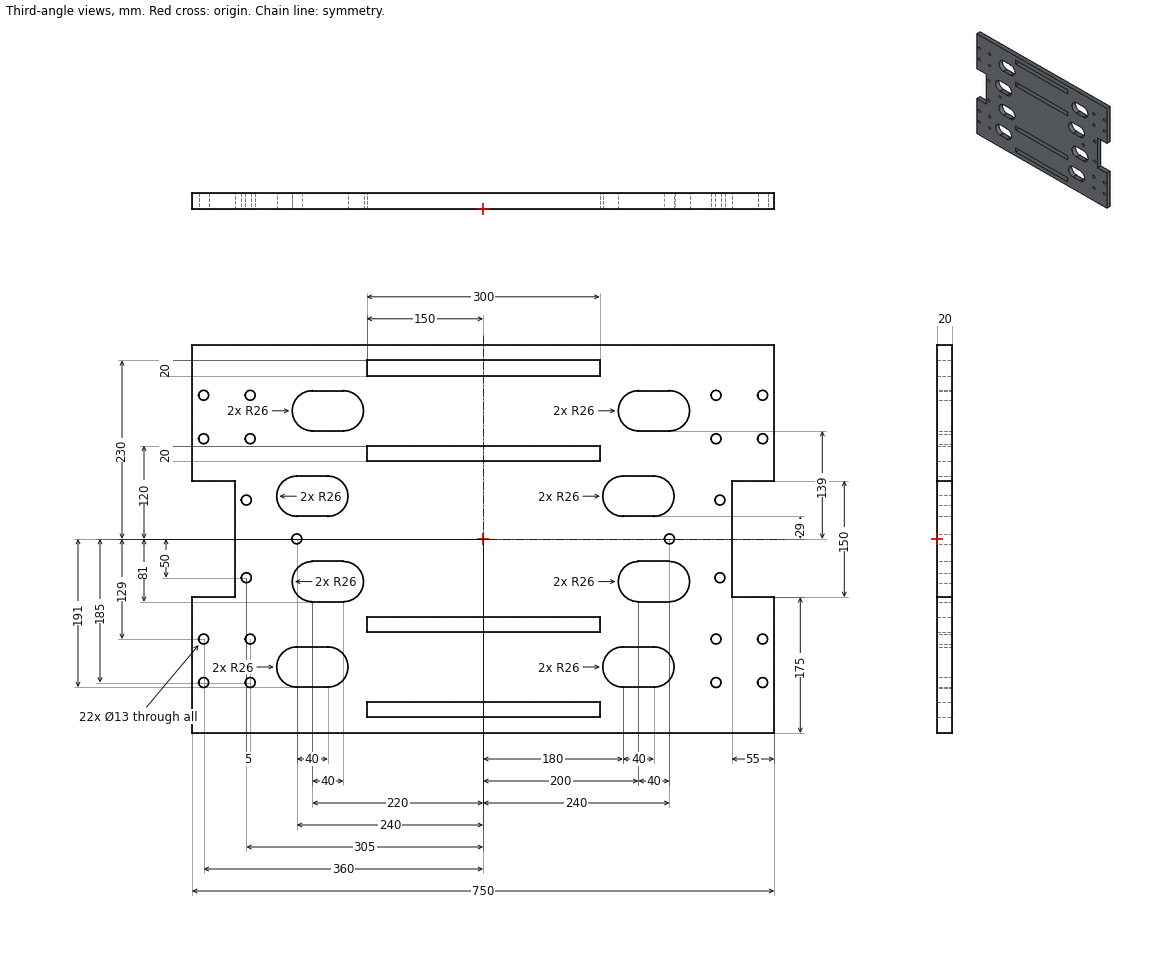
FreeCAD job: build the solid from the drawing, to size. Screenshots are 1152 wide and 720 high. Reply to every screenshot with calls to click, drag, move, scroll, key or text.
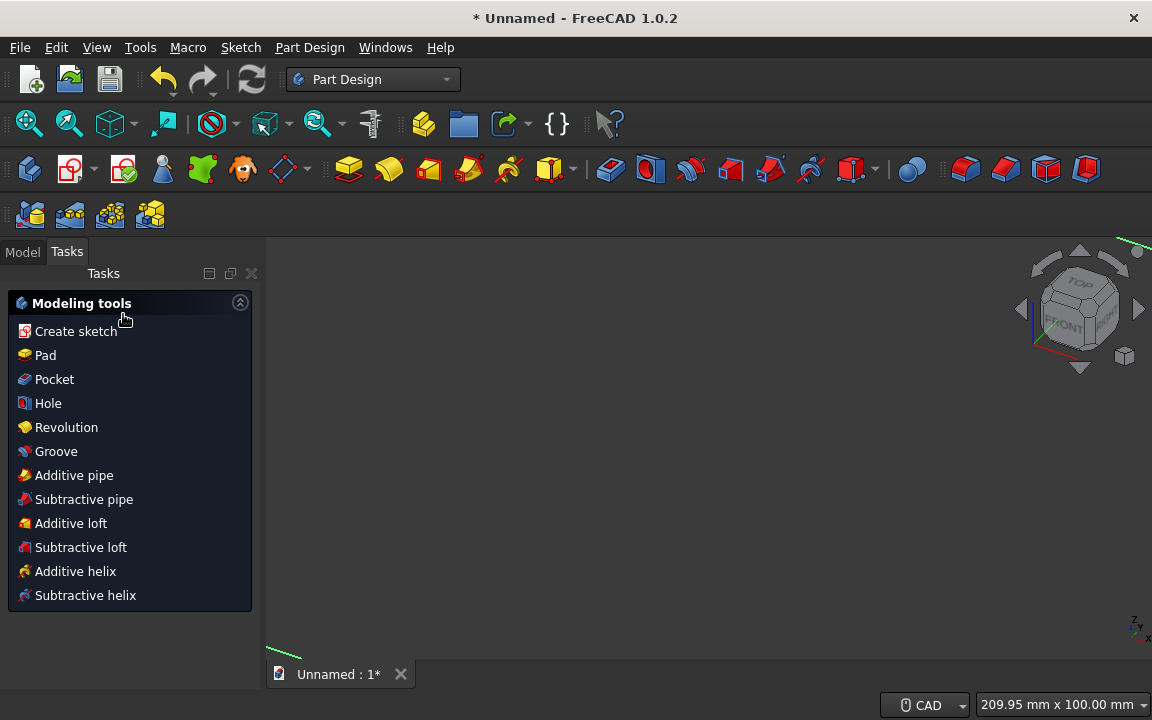
click(350, 170)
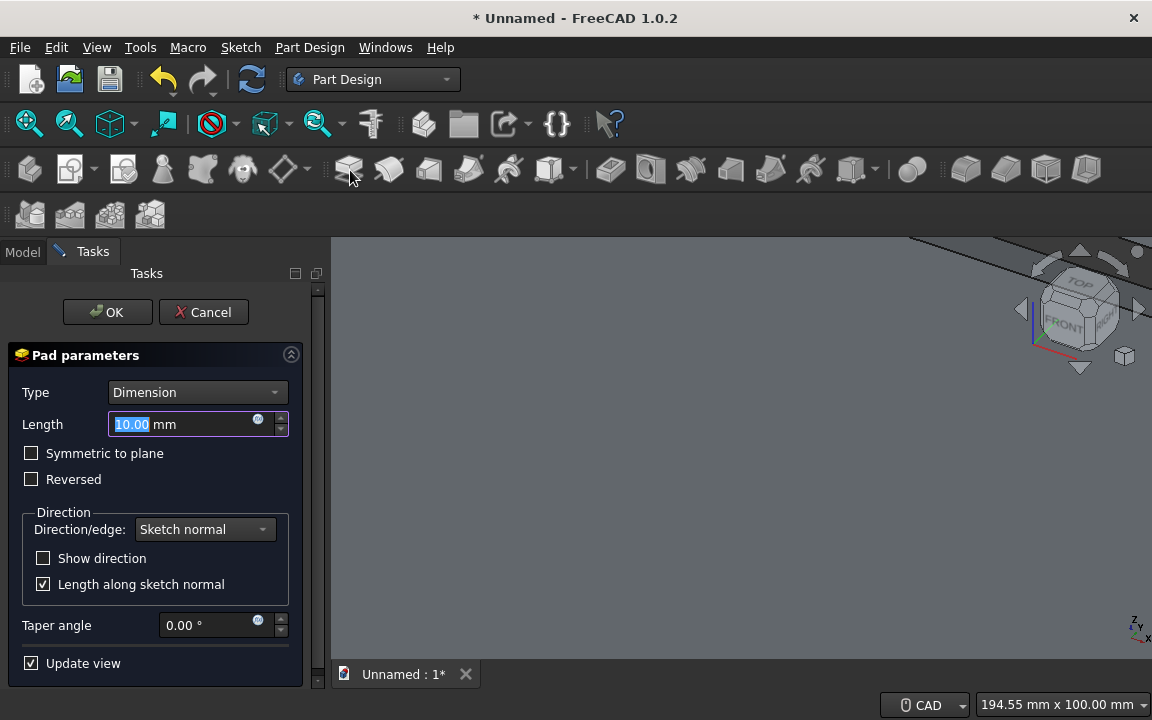
text(20)
key(Tab)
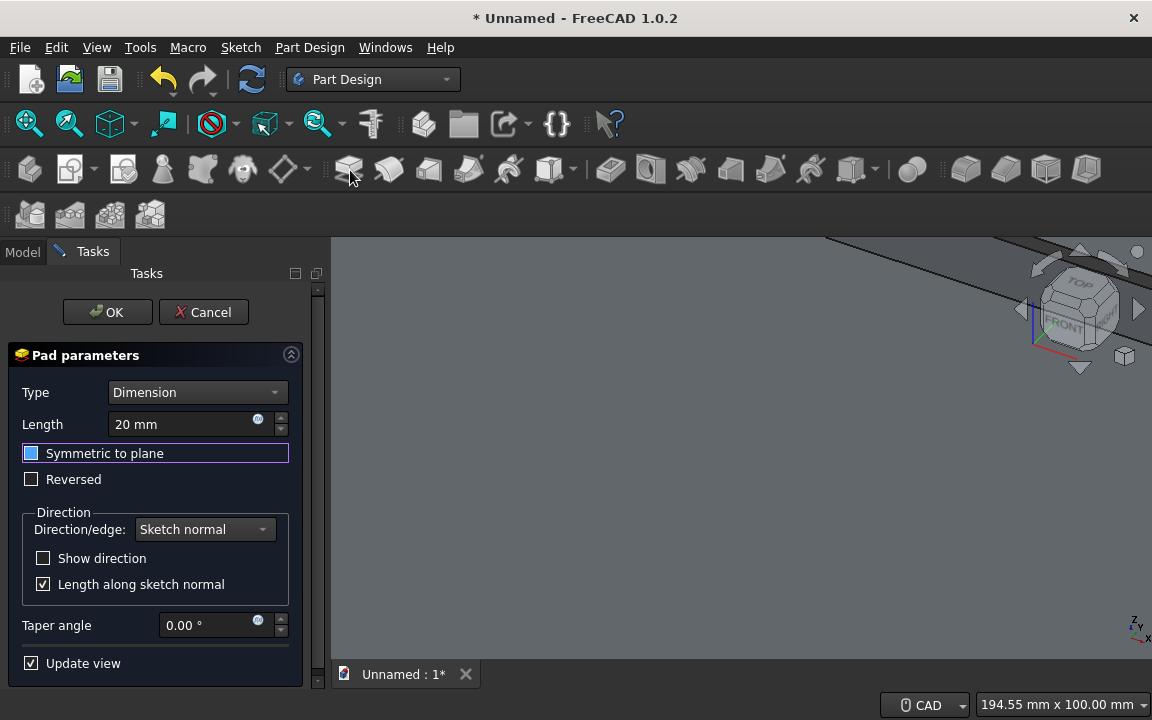
click(30, 479)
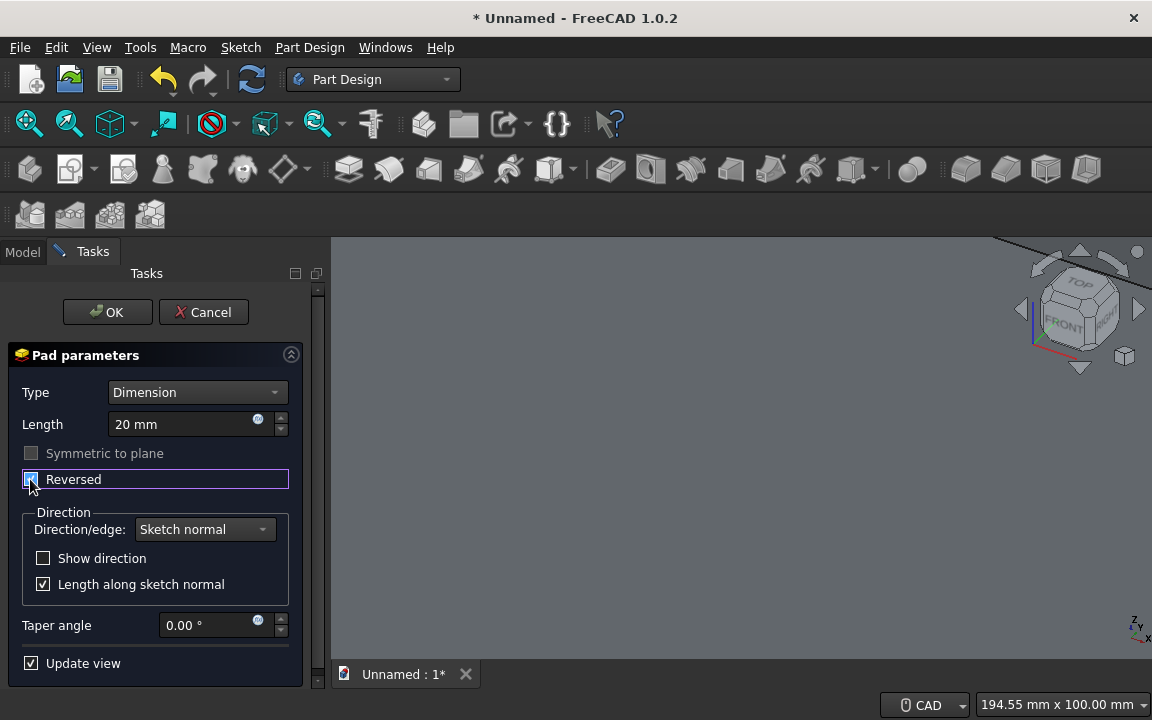
click(108, 312)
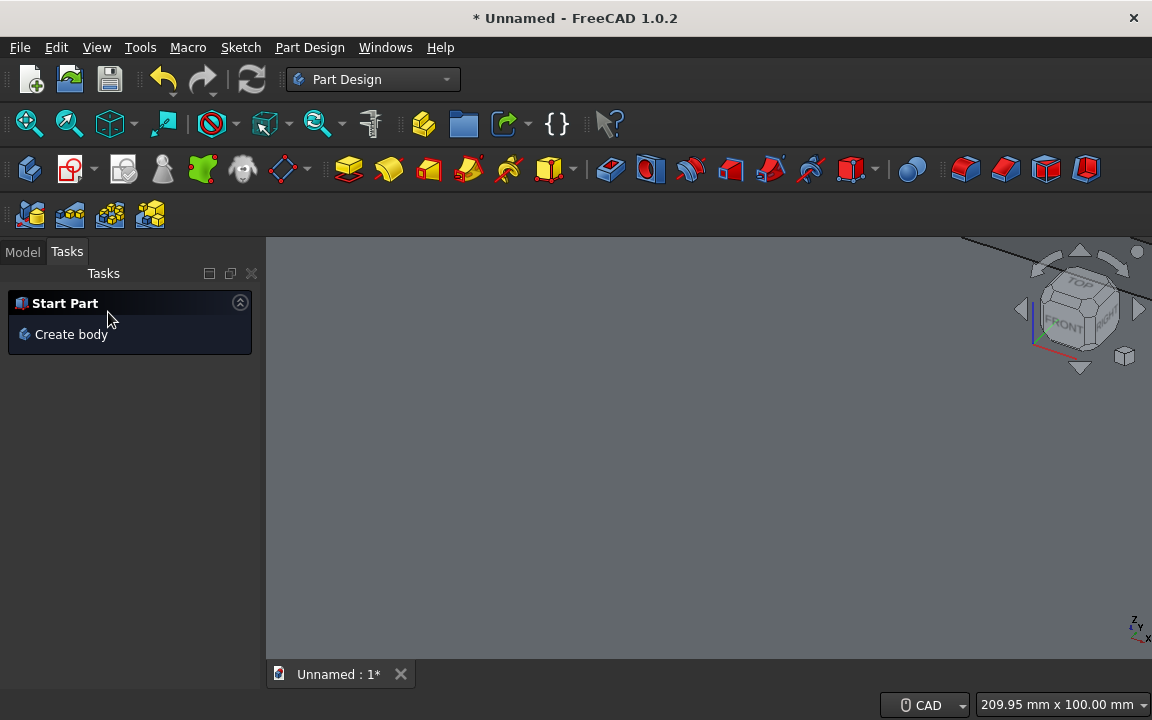
click(30, 124)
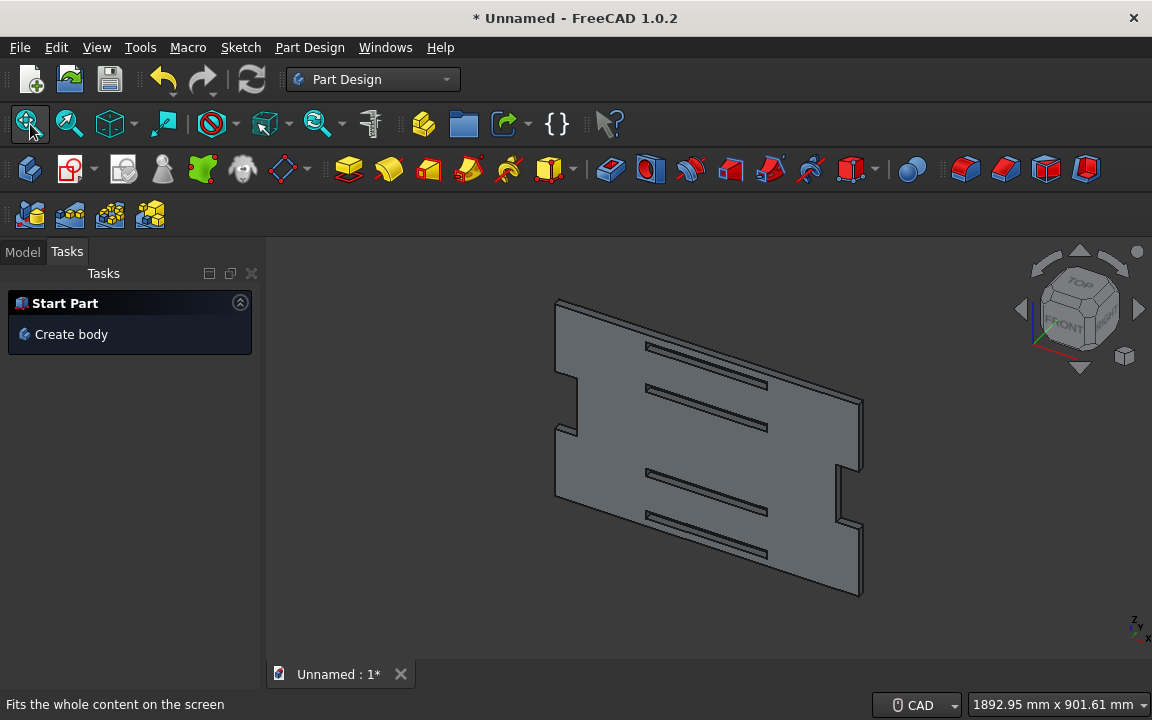
key(4)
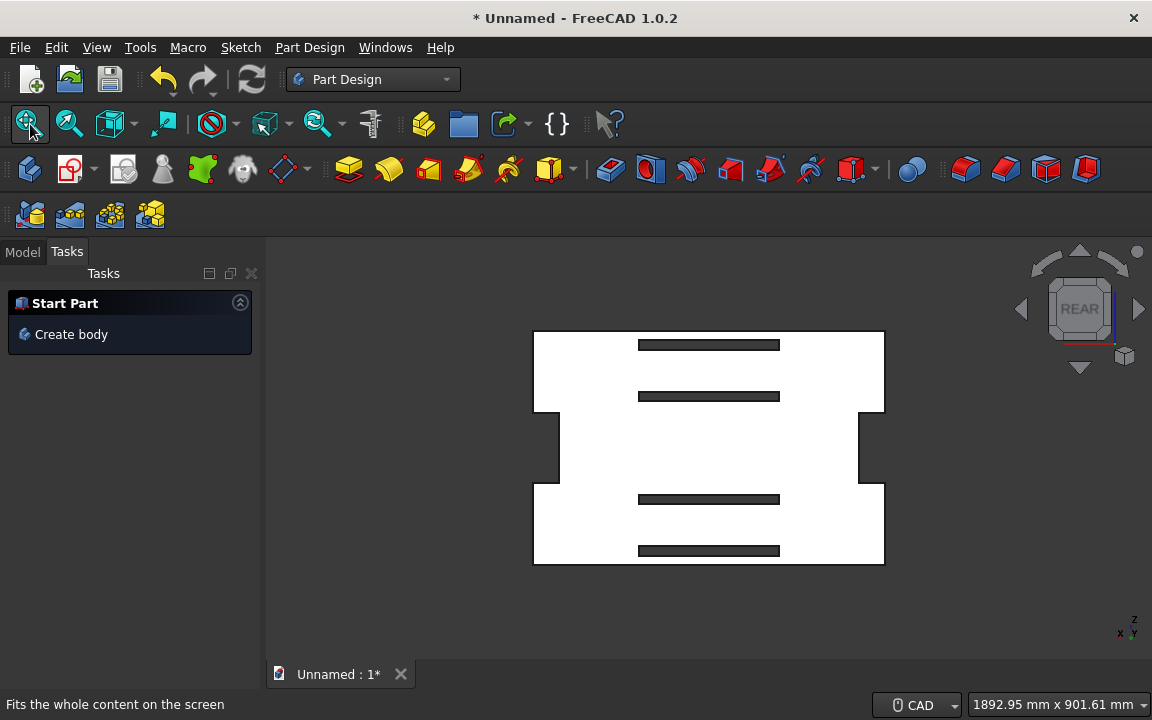
click(809, 447)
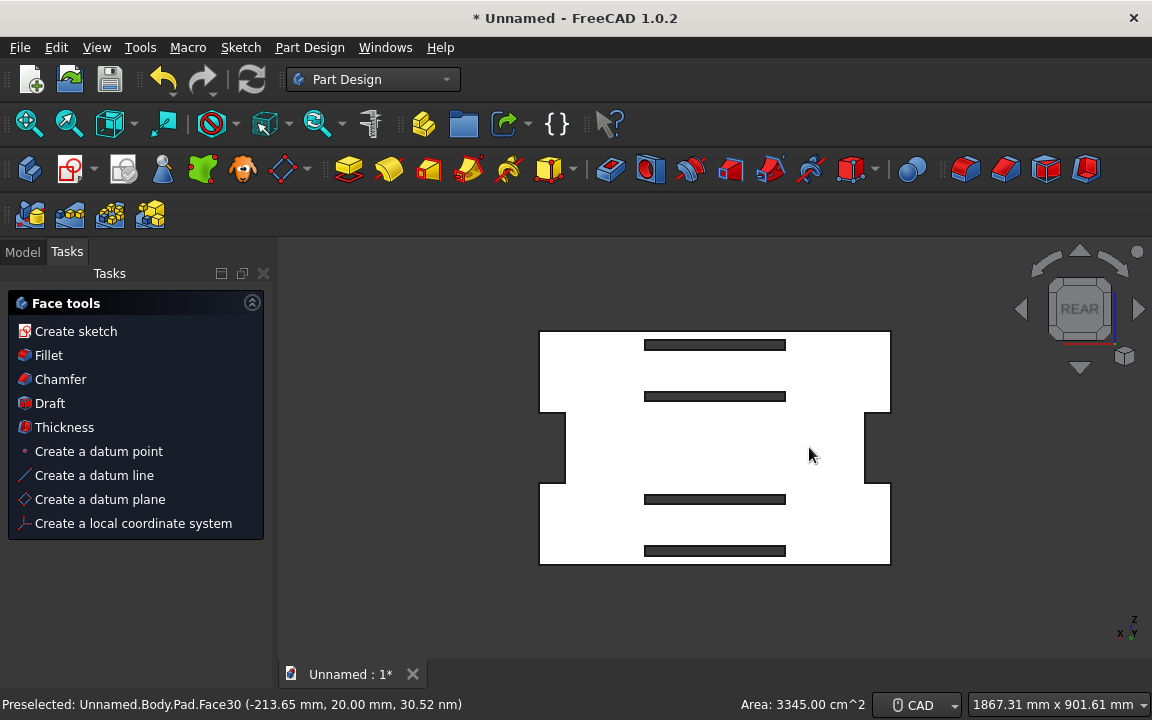
click(70, 170)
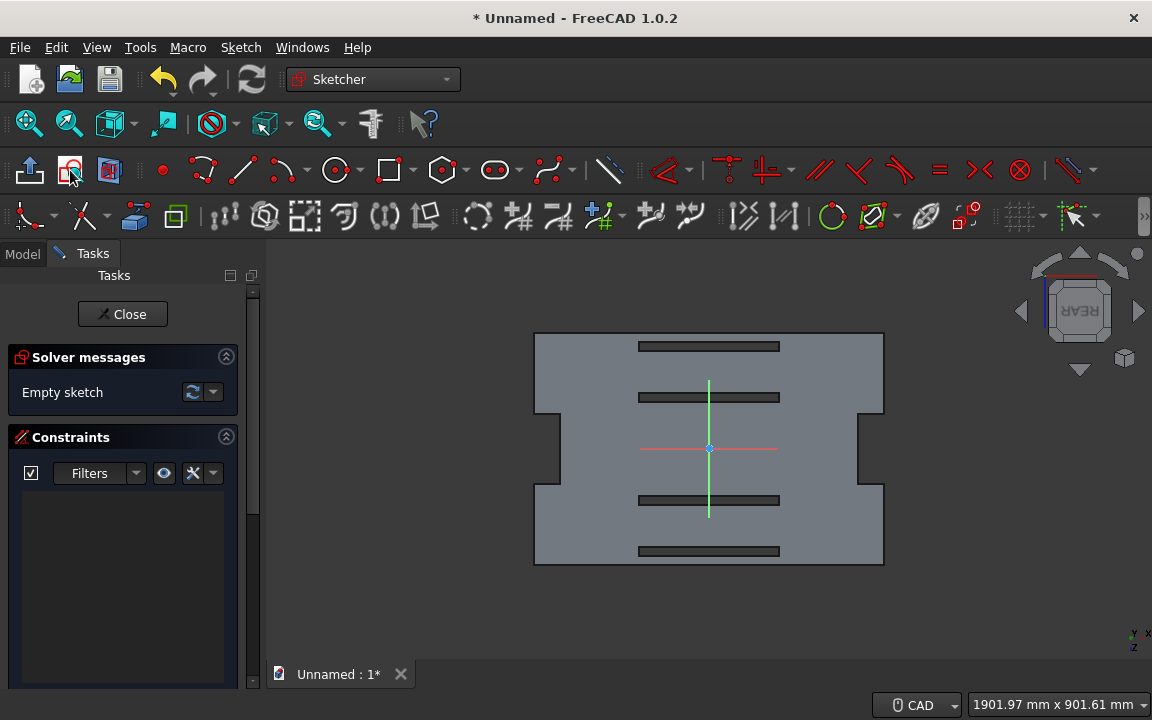
scroll(848, 449, up, 2)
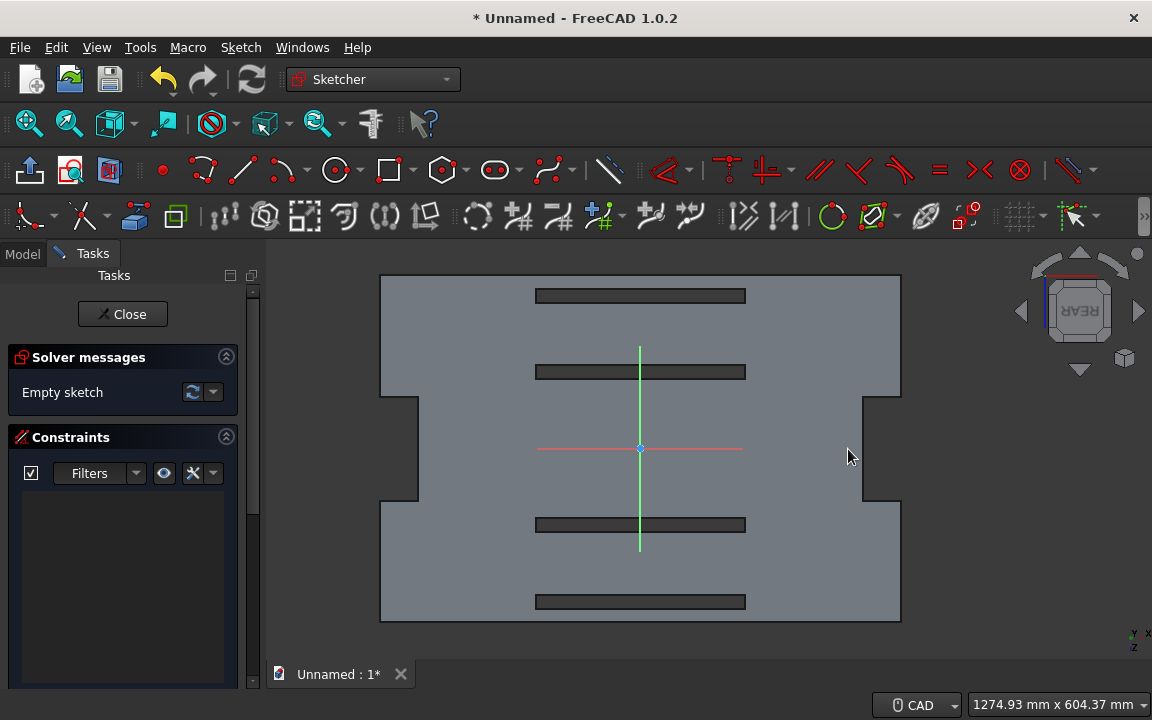
click(336, 170)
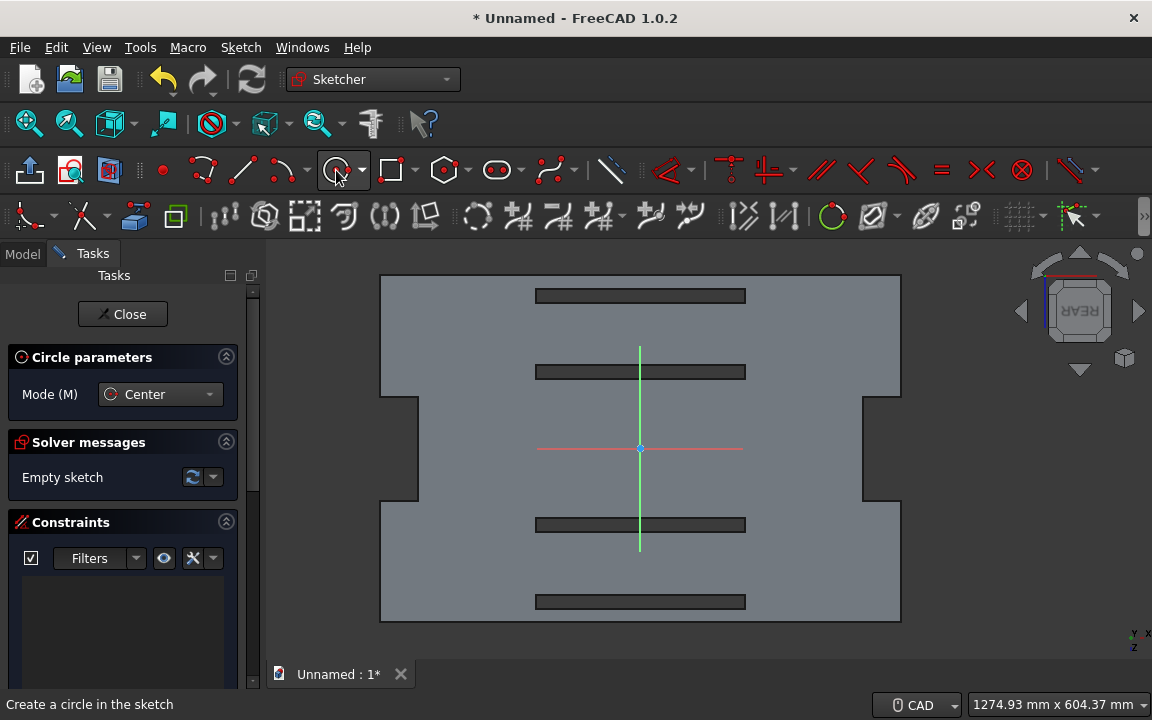
scroll(390, 359, up, 9)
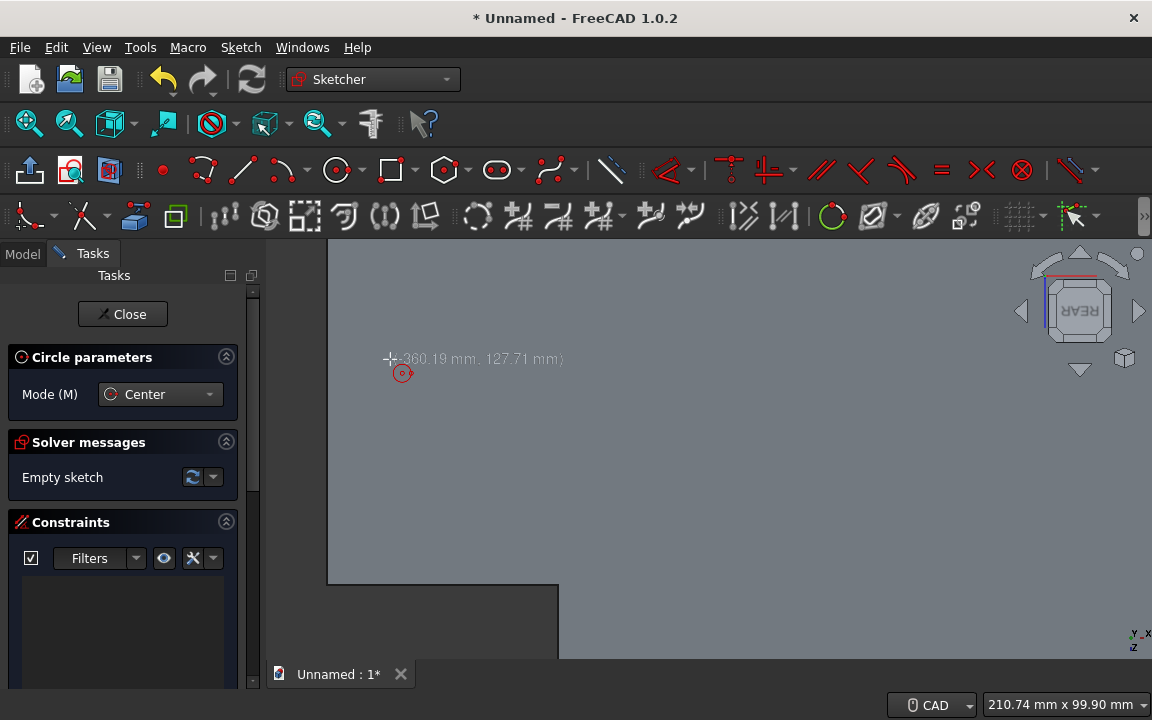
scroll(390, 360, down, 9)